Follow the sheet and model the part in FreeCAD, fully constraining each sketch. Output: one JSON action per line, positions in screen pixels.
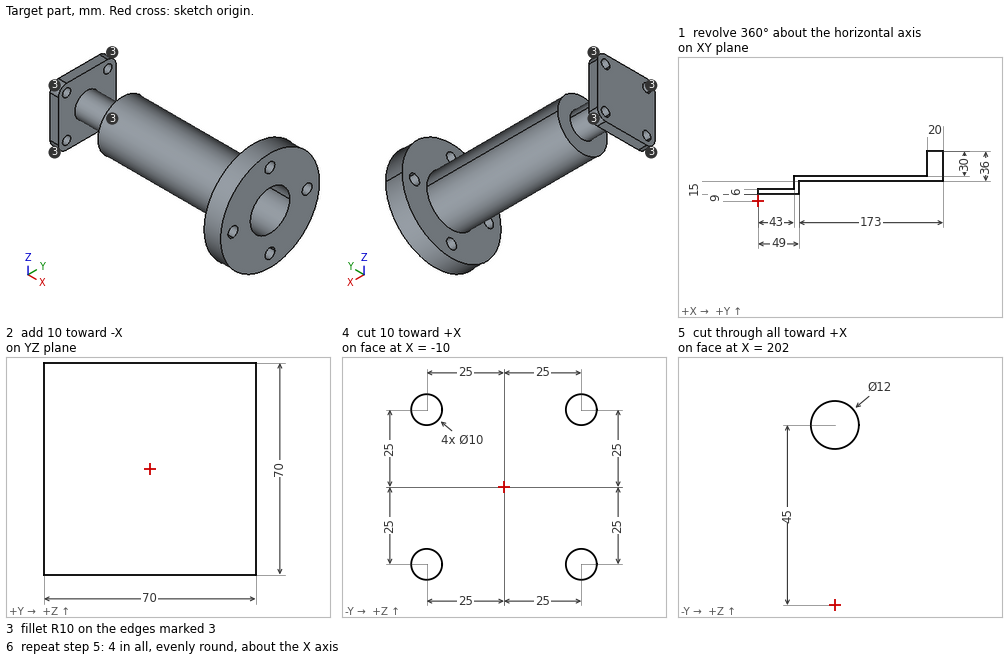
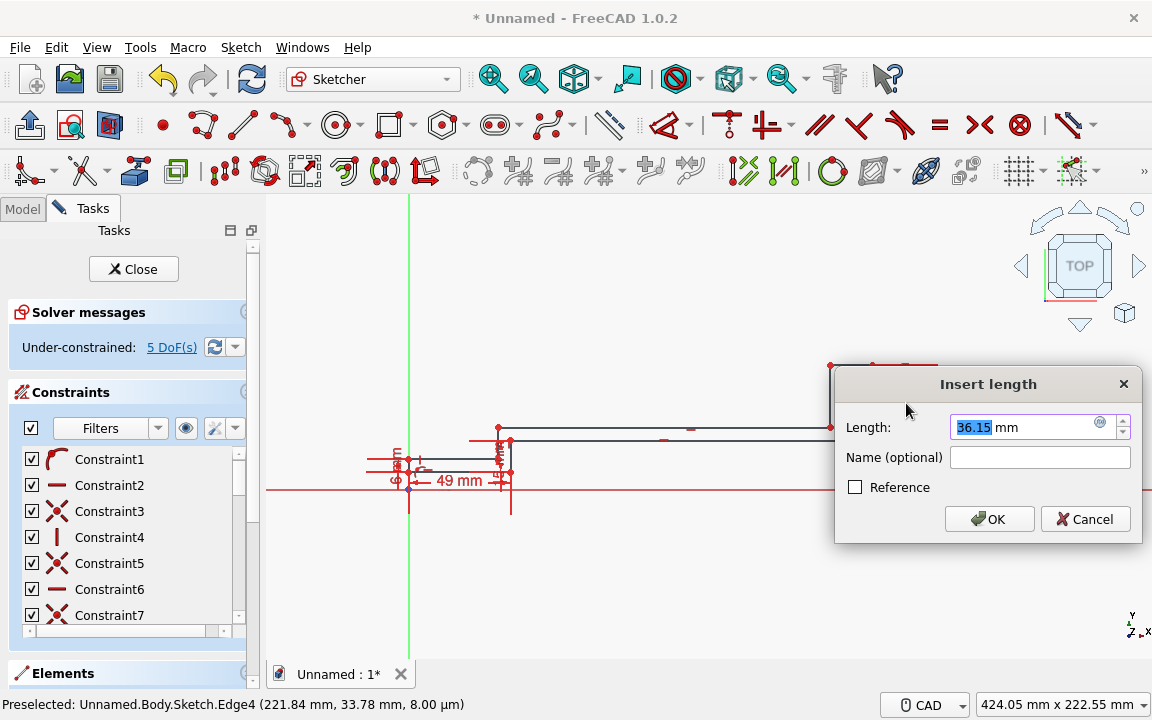
{"action": "type", "text": "36"}
{"action": "key", "text": "Return"}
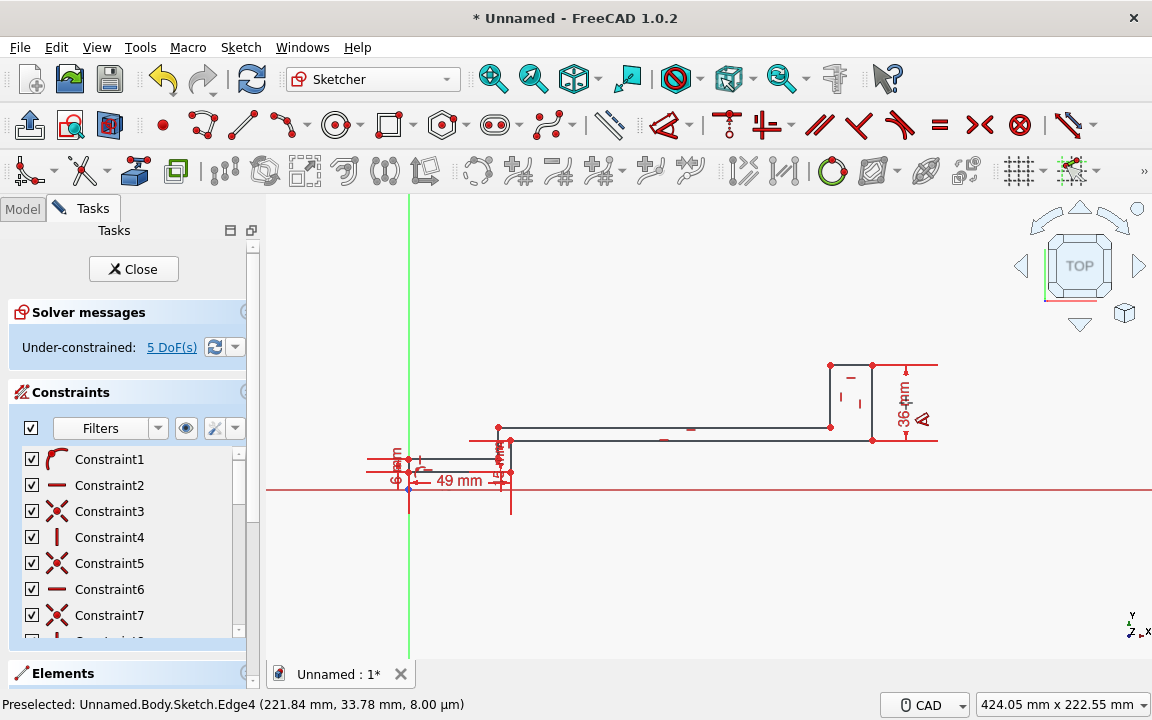
{"action": "left_click", "coordinate": [860, 365]}
{"action": "left_click", "coordinate": [851, 331]}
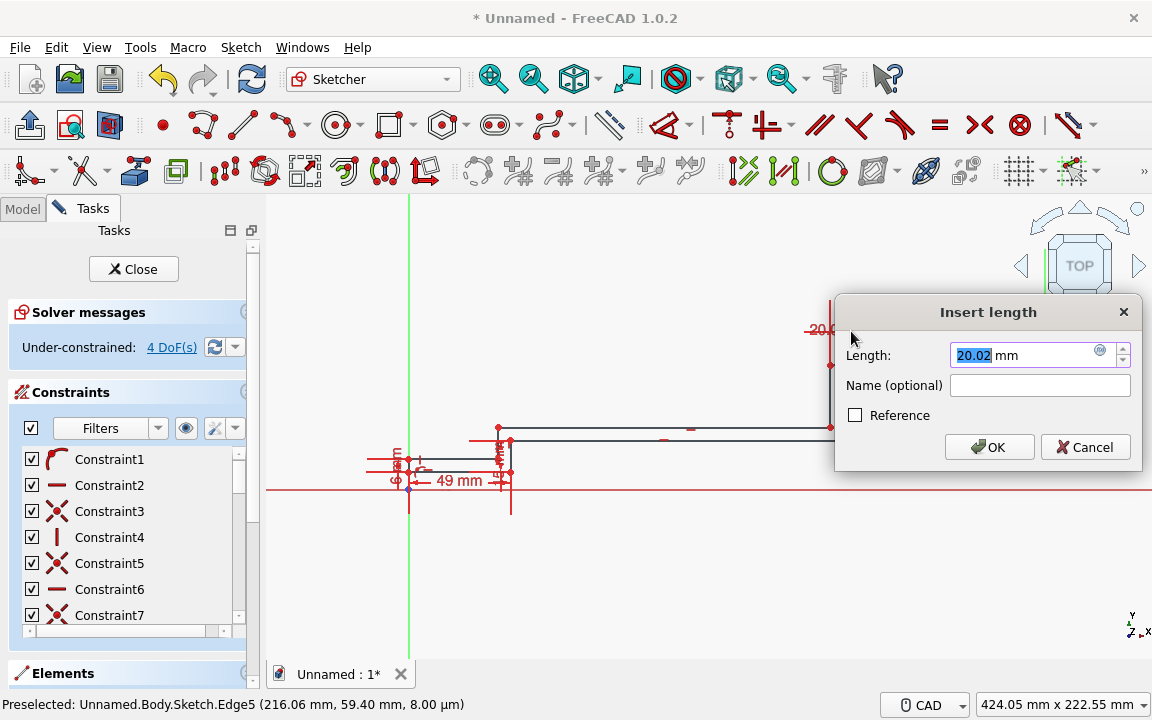
{"action": "type", "text": "20"}
{"action": "key", "text": "Return"}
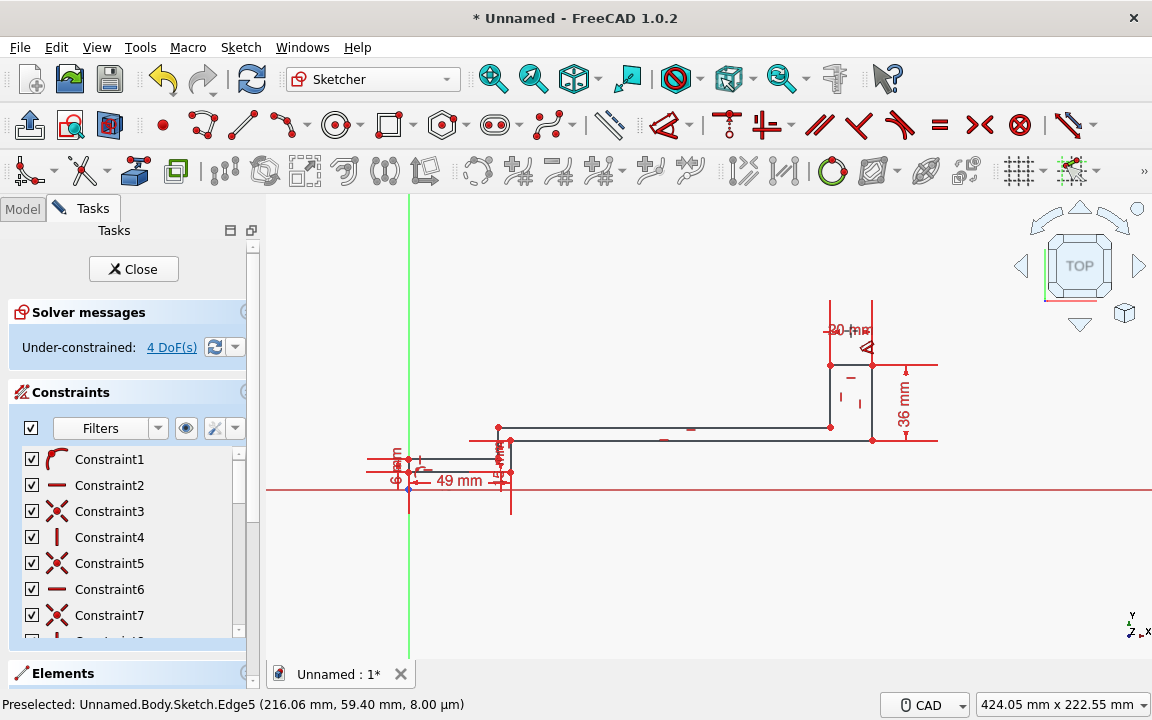
{"action": "left_click", "coordinate": [830, 384]}
{"action": "left_click", "coordinate": [796, 397]}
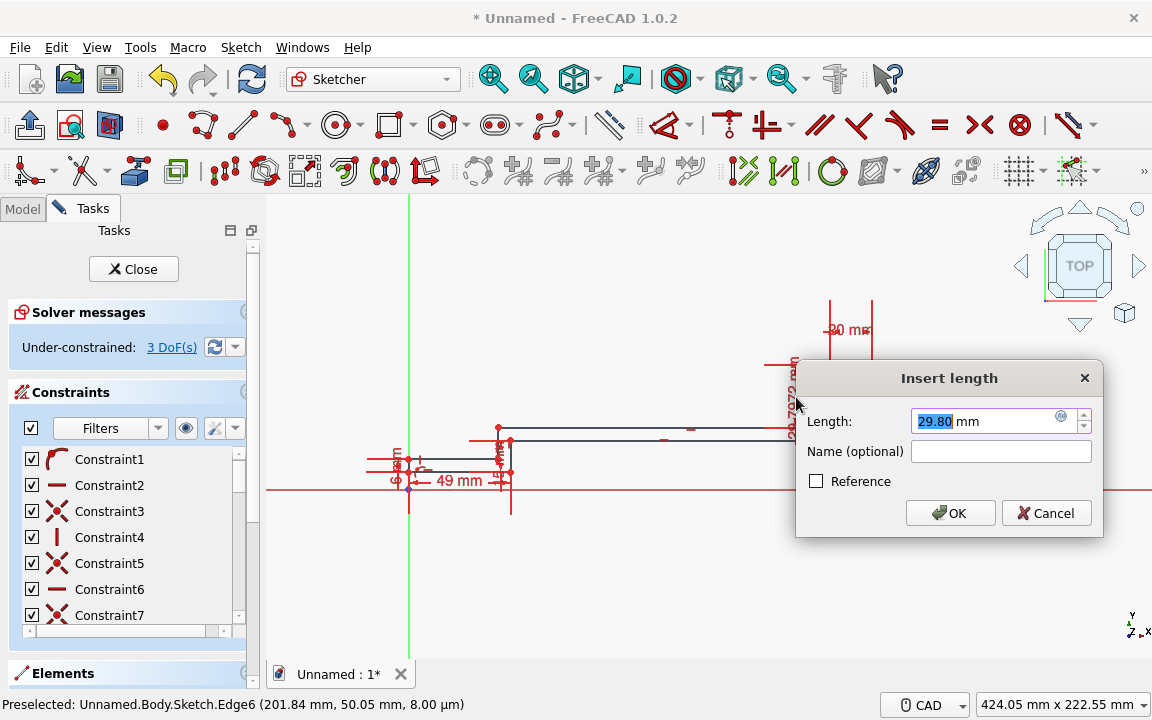
{"action": "type", "text": "30"}
{"action": "key", "text": "Return"}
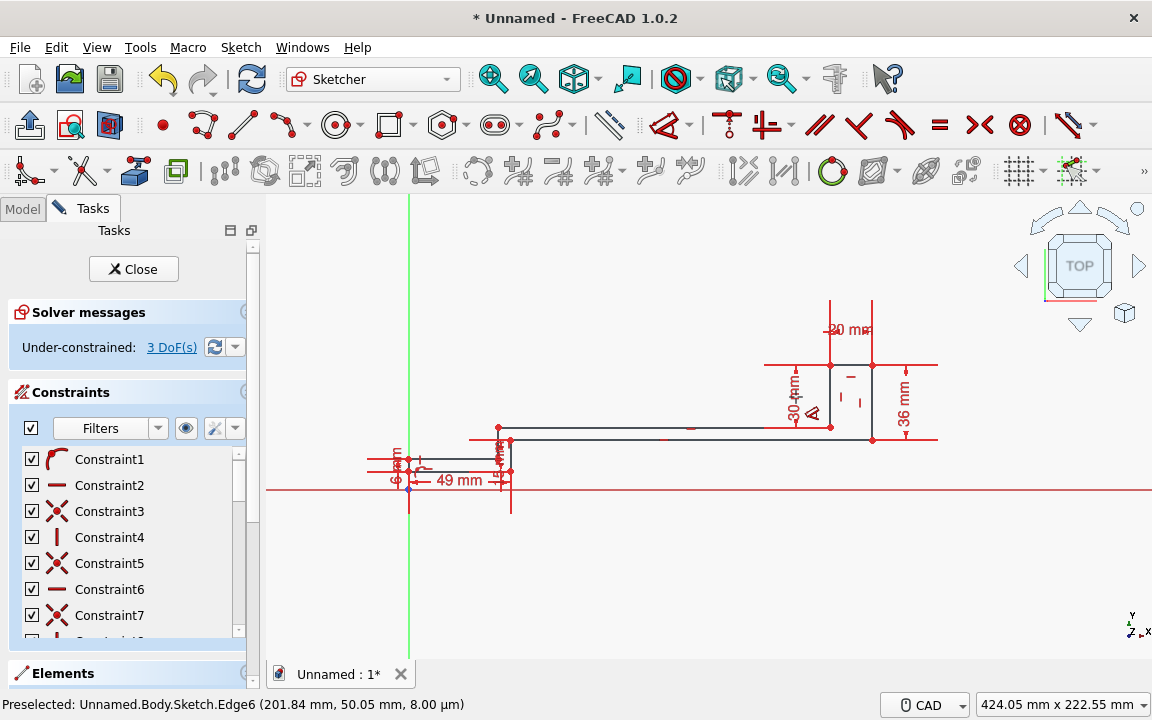
{"action": "left_click", "coordinate": [471, 459]}
{"action": "left_click", "coordinate": [453, 425]}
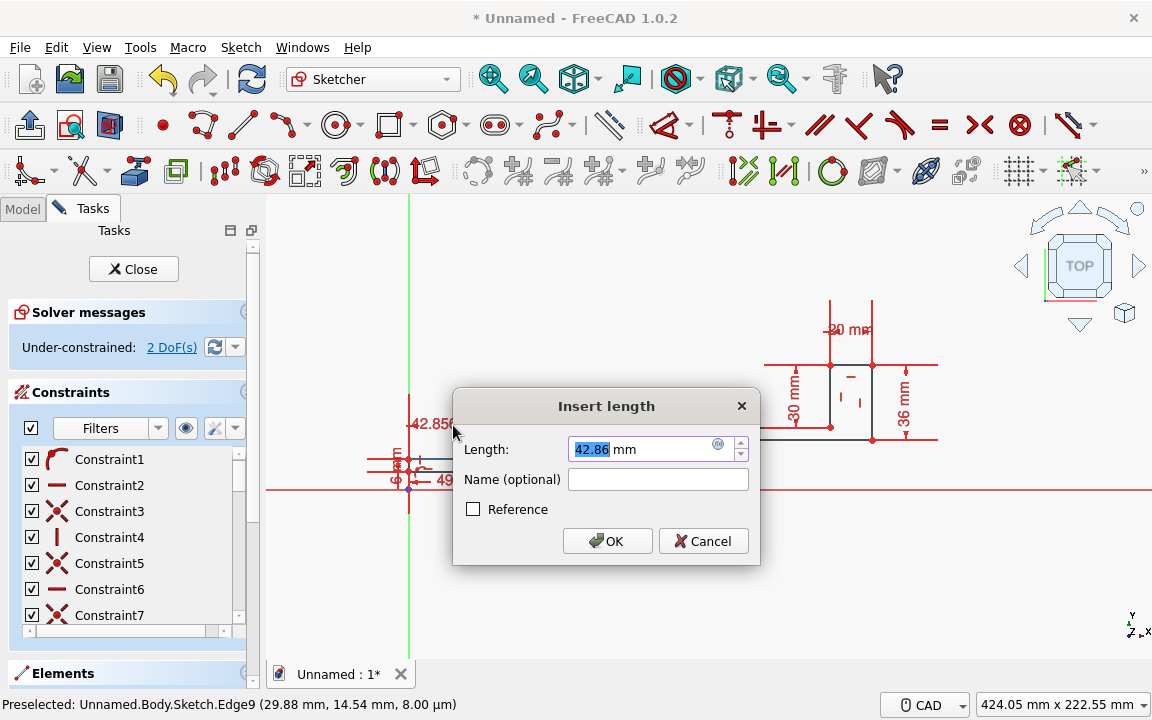
{"action": "type", "text": "43"}
{"action": "key", "text": "Return"}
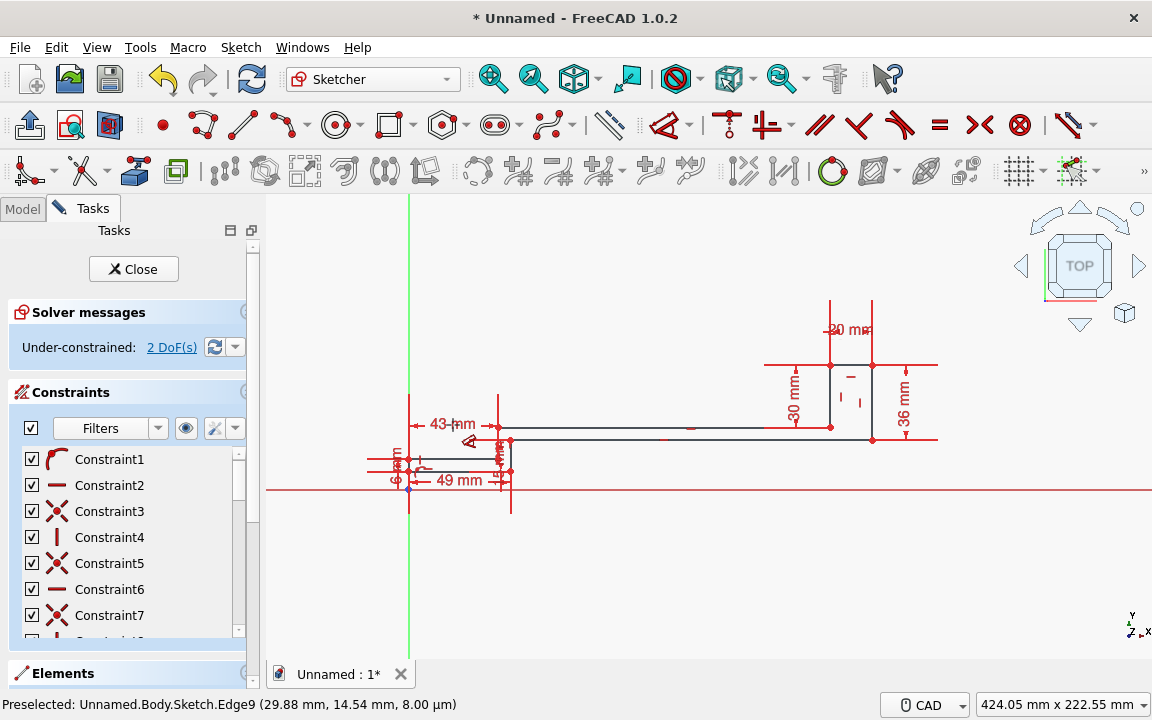
{"action": "scroll", "coordinate": [409, 472], "scroll_direction": "up", "scroll_amount": 4}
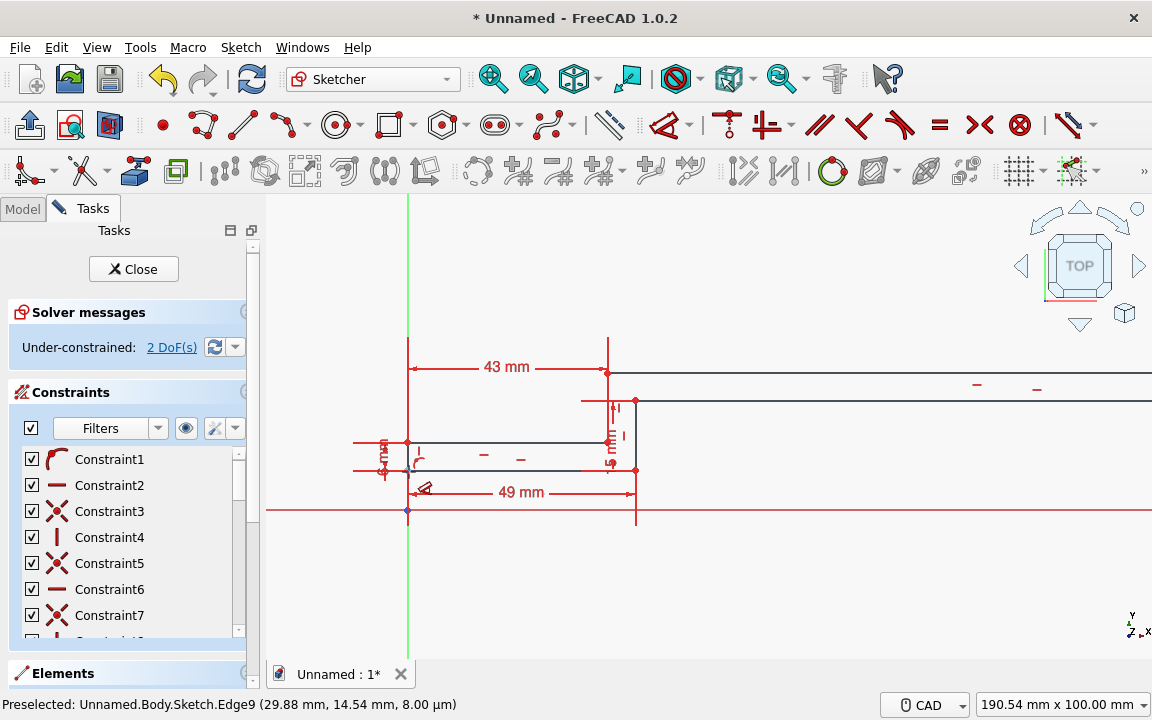
{"action": "left_click", "coordinate": [408, 471]}
{"action": "left_click", "coordinate": [374, 491]}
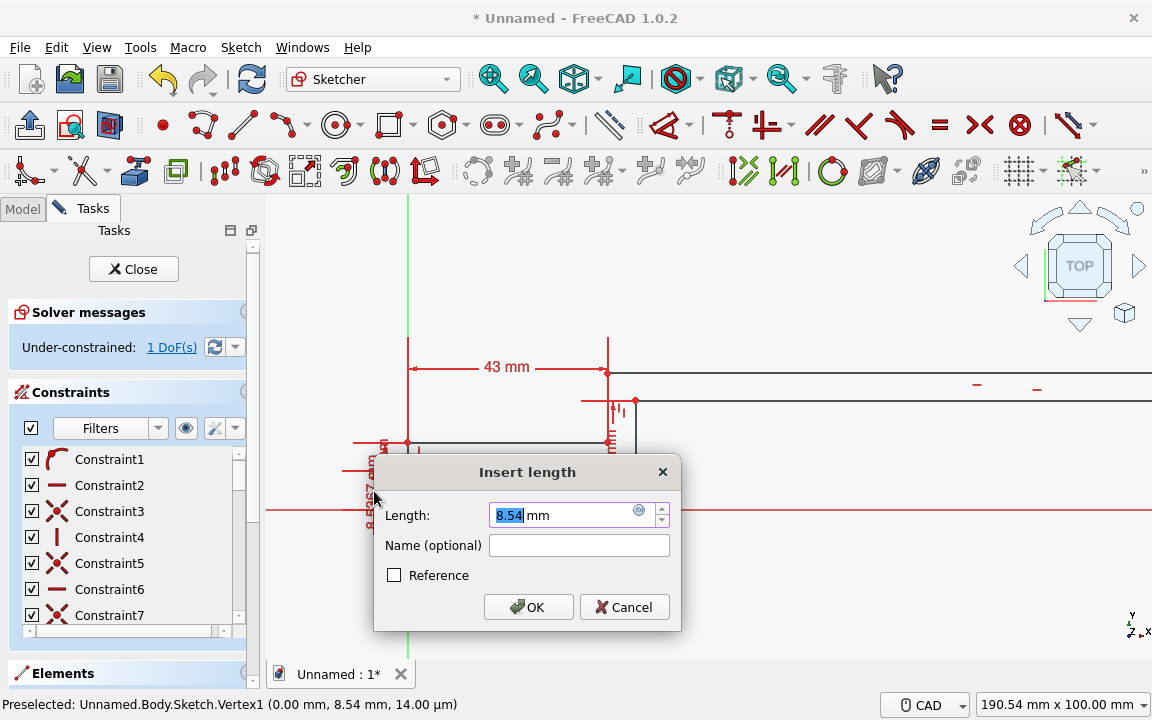
{"action": "type", "text": "9"}
{"action": "key", "text": "Return"}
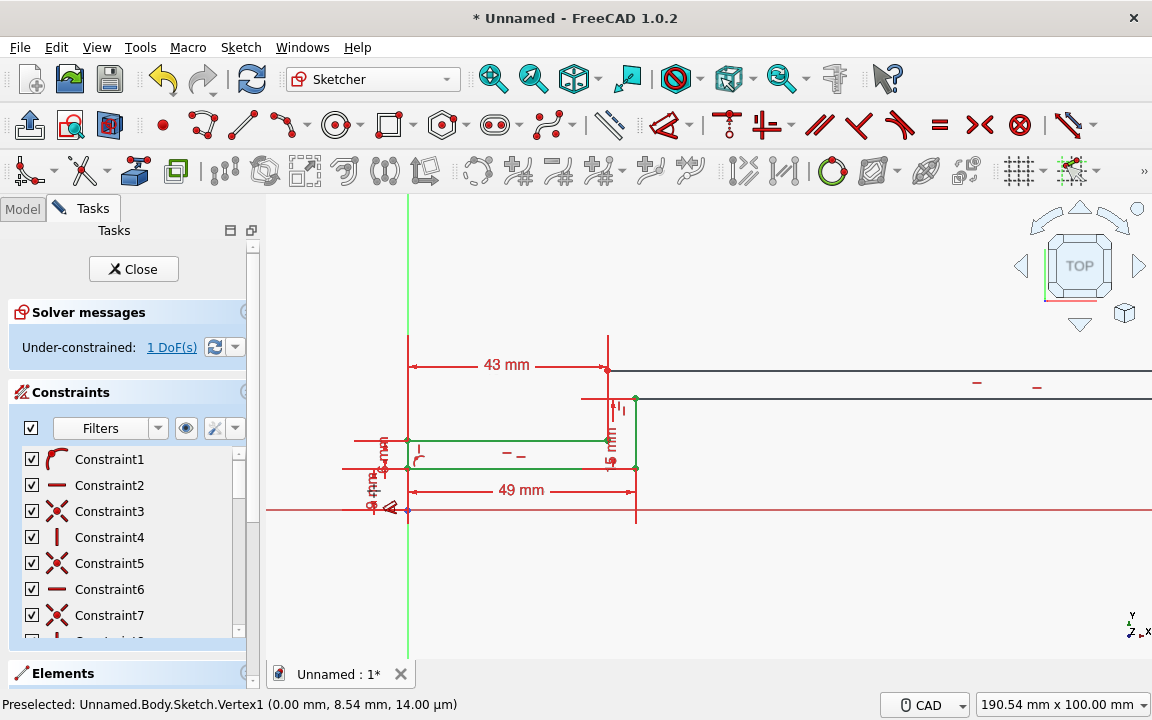
{"action": "left_click", "coordinate": [877, 399]}
{"action": "left_click", "coordinate": [811, 433]}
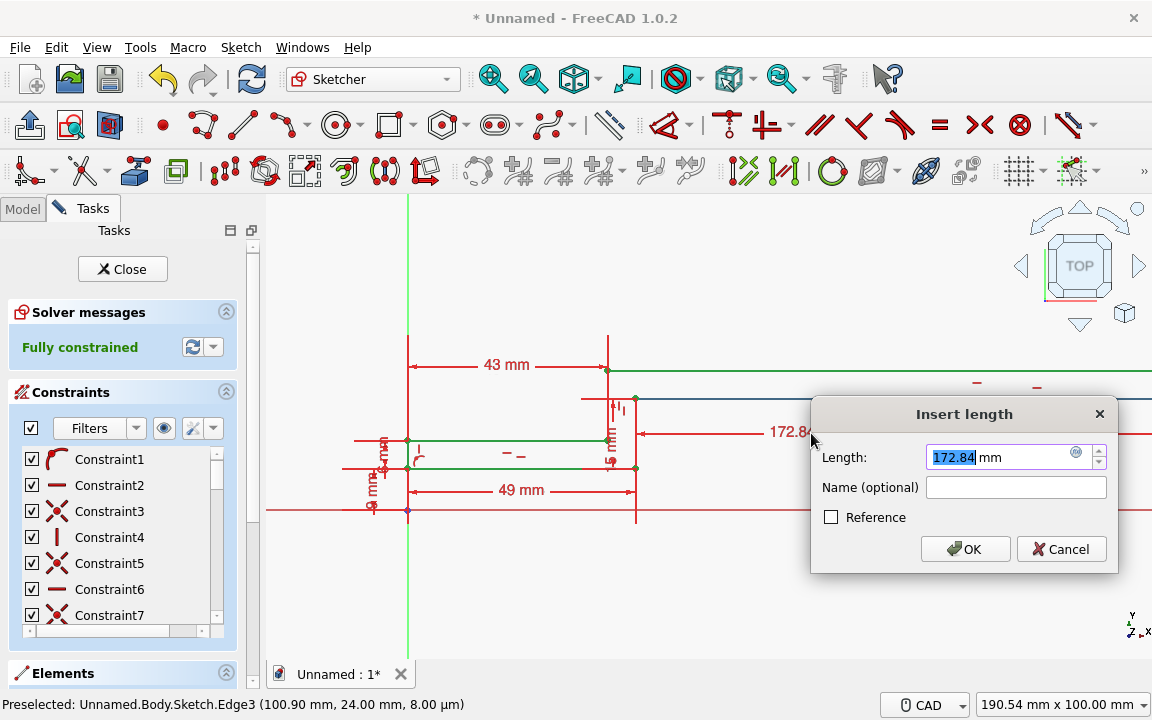
{"action": "type", "text": "173"}
{"action": "key", "text": "Return"}
{"action": "key", "text": "Escape"}